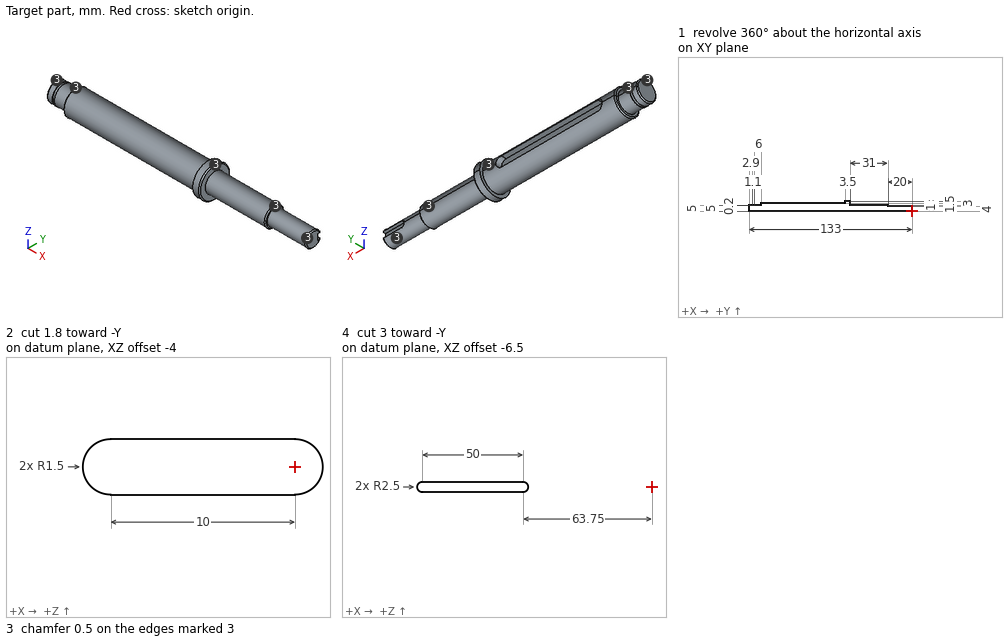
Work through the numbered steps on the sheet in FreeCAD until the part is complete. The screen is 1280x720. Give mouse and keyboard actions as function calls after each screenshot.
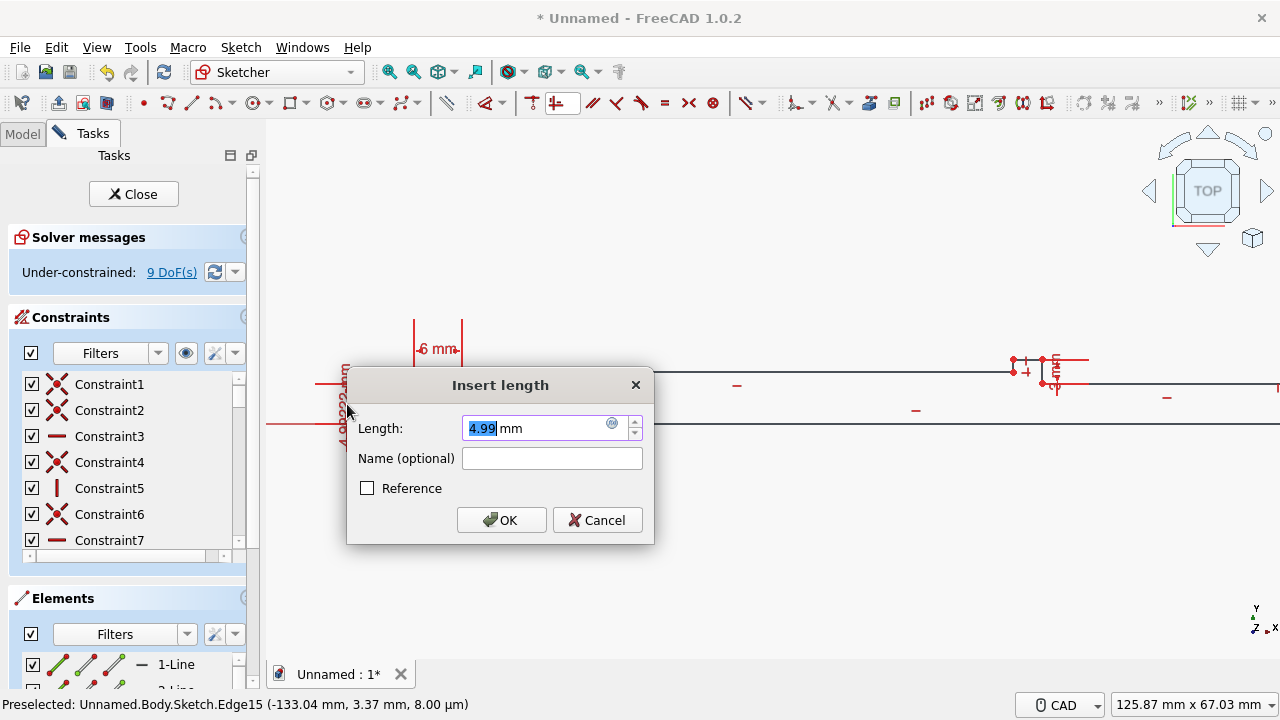
text(5)
key(Return)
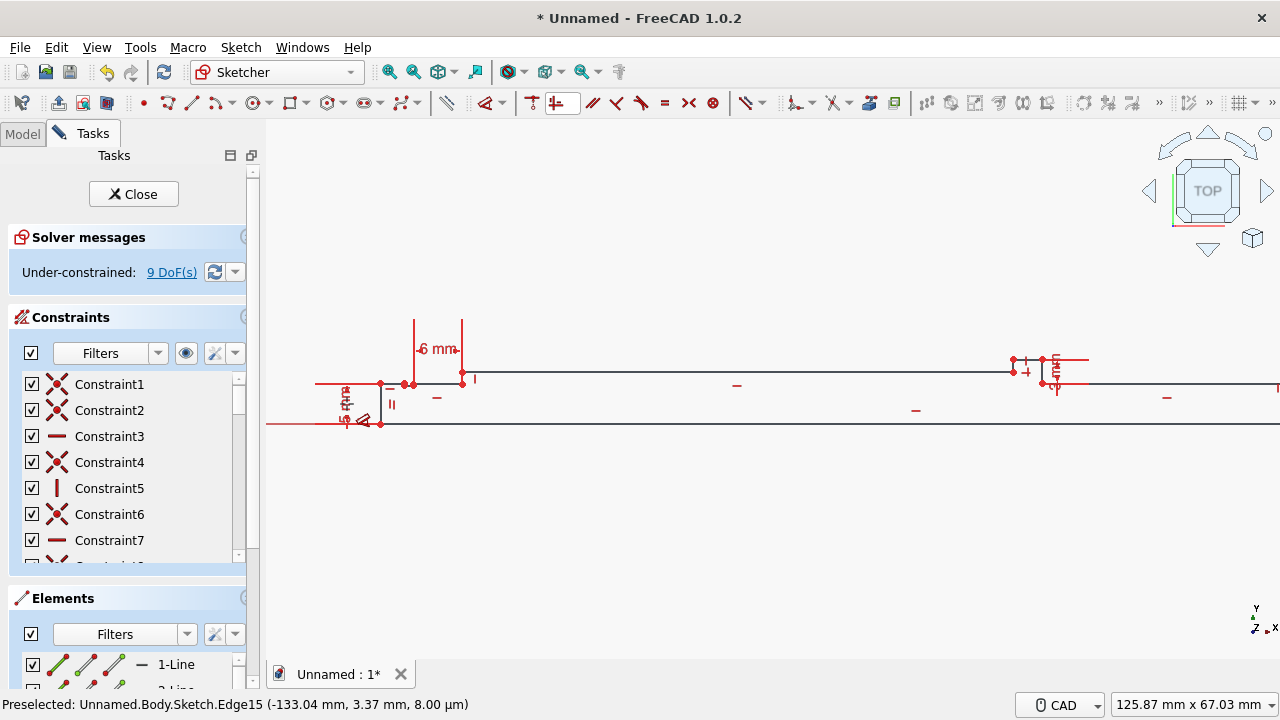
scroll(446, 385, down, 3)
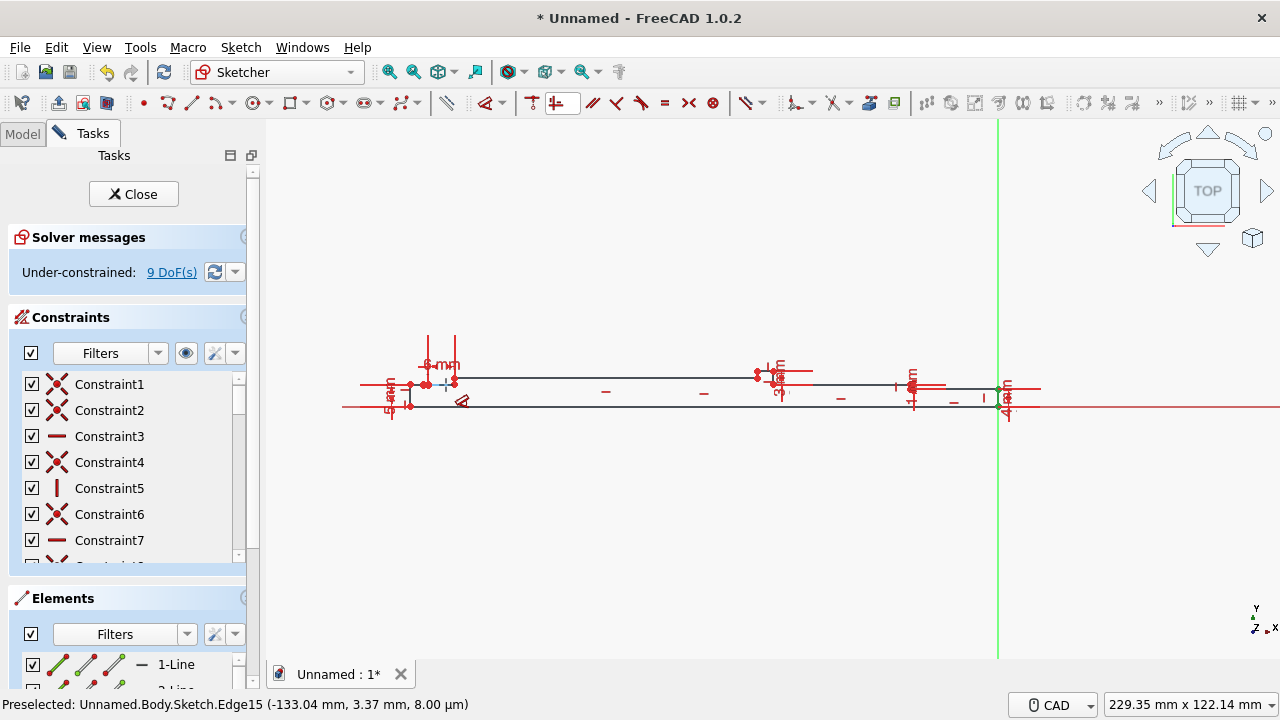
click(972, 389)
click(954, 423)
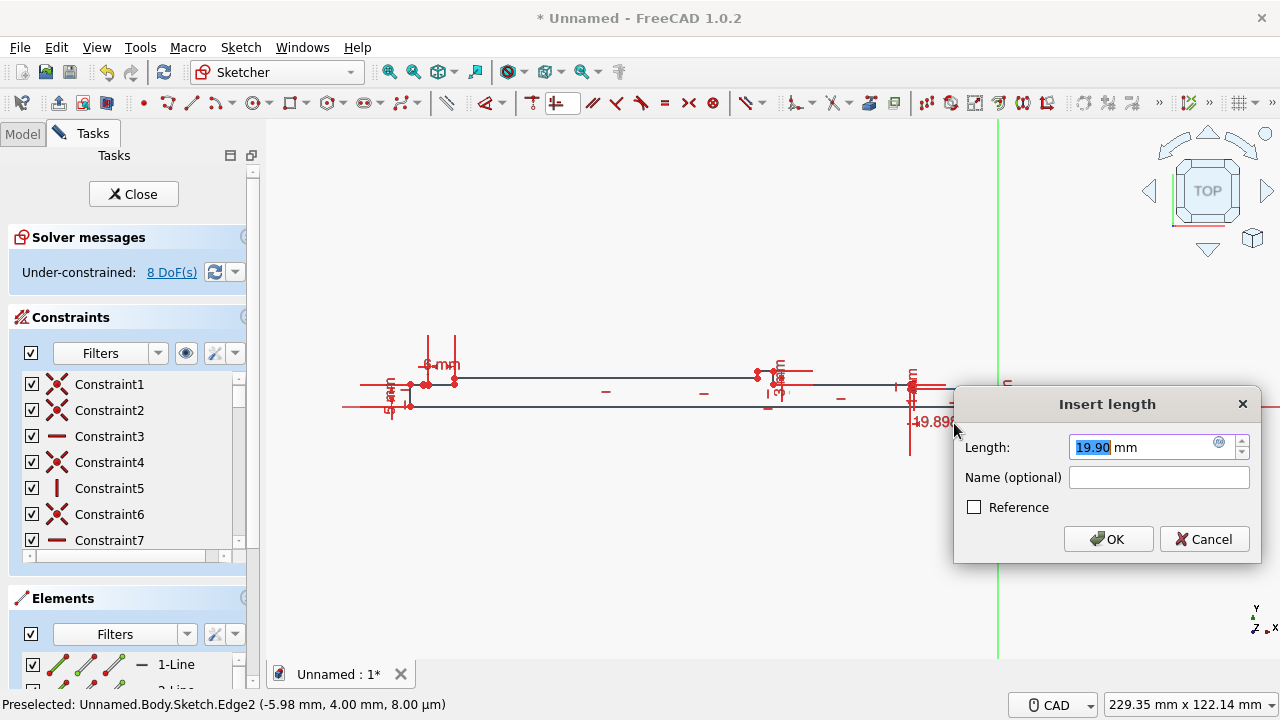
text(20)
key(Return)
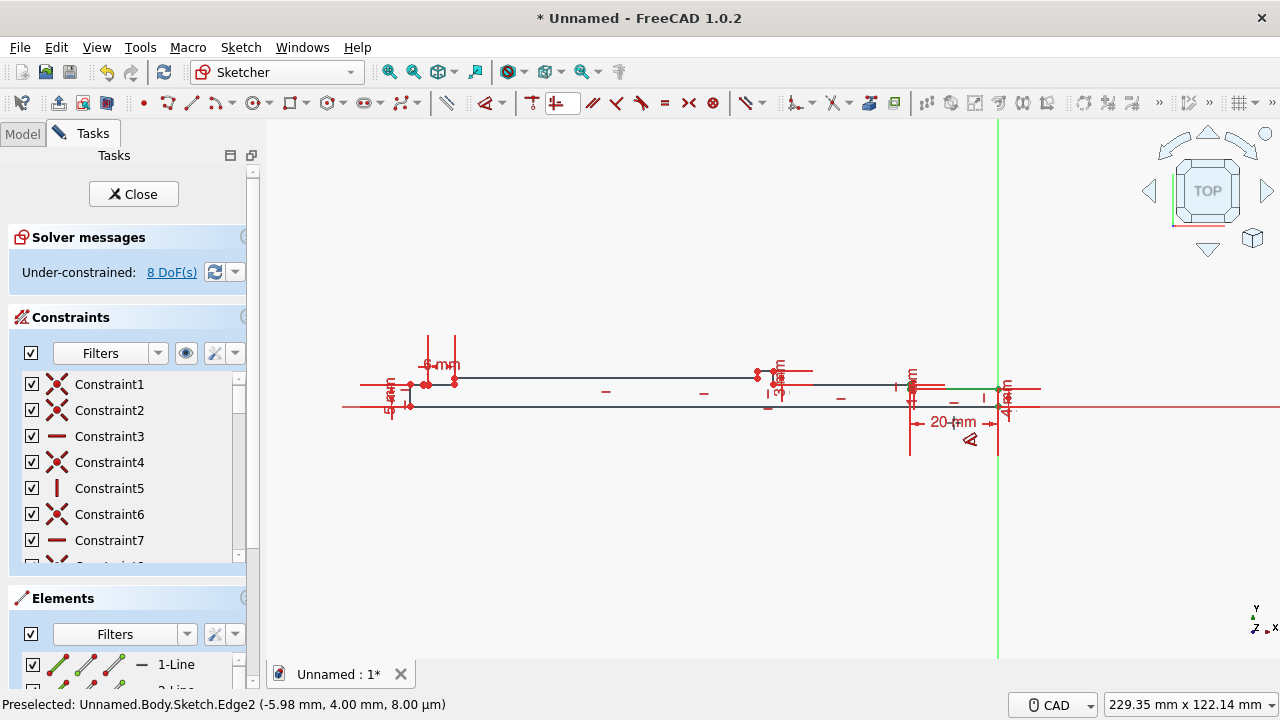
click(869, 385)
click(842, 351)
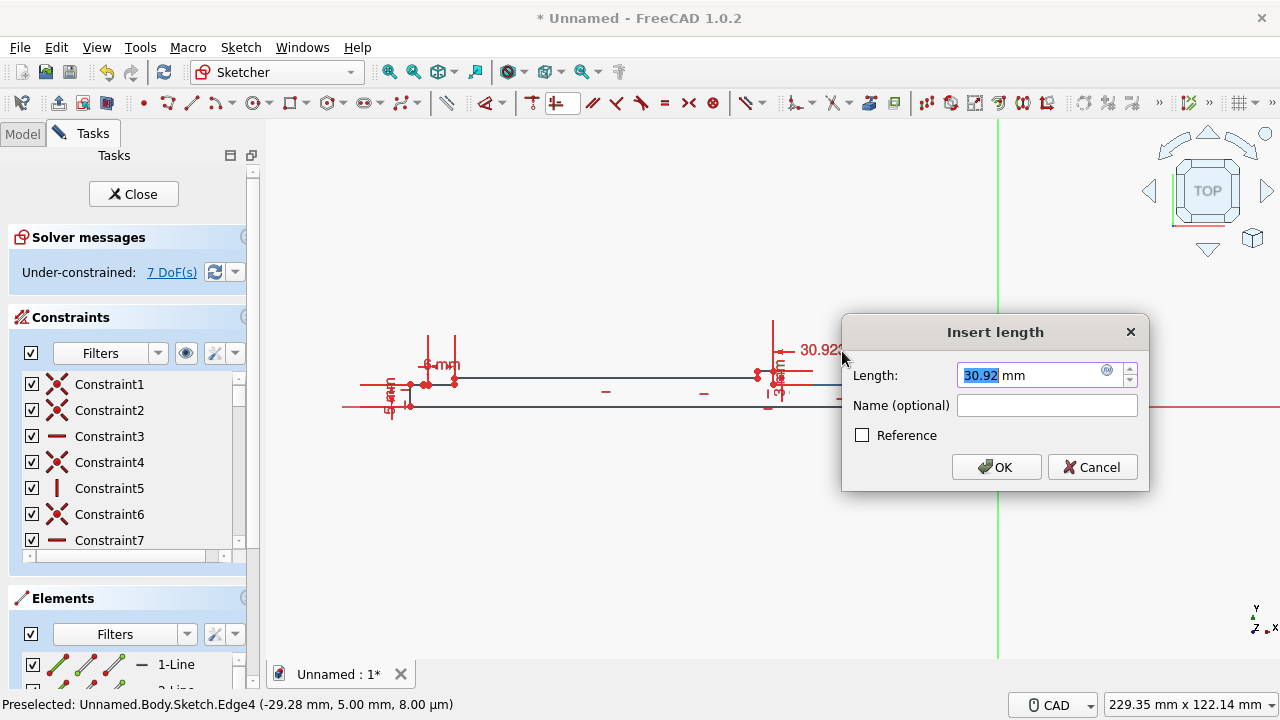
text(31)
key(Return)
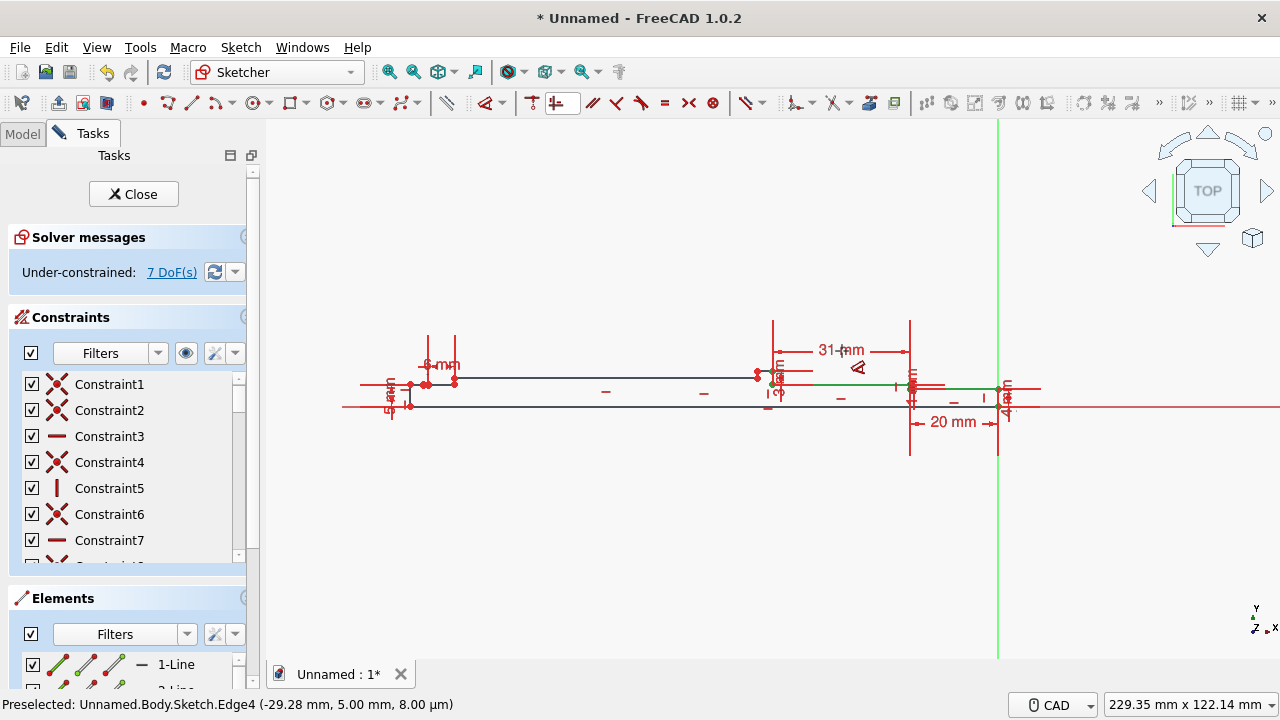
scroll(455, 385, up, 4)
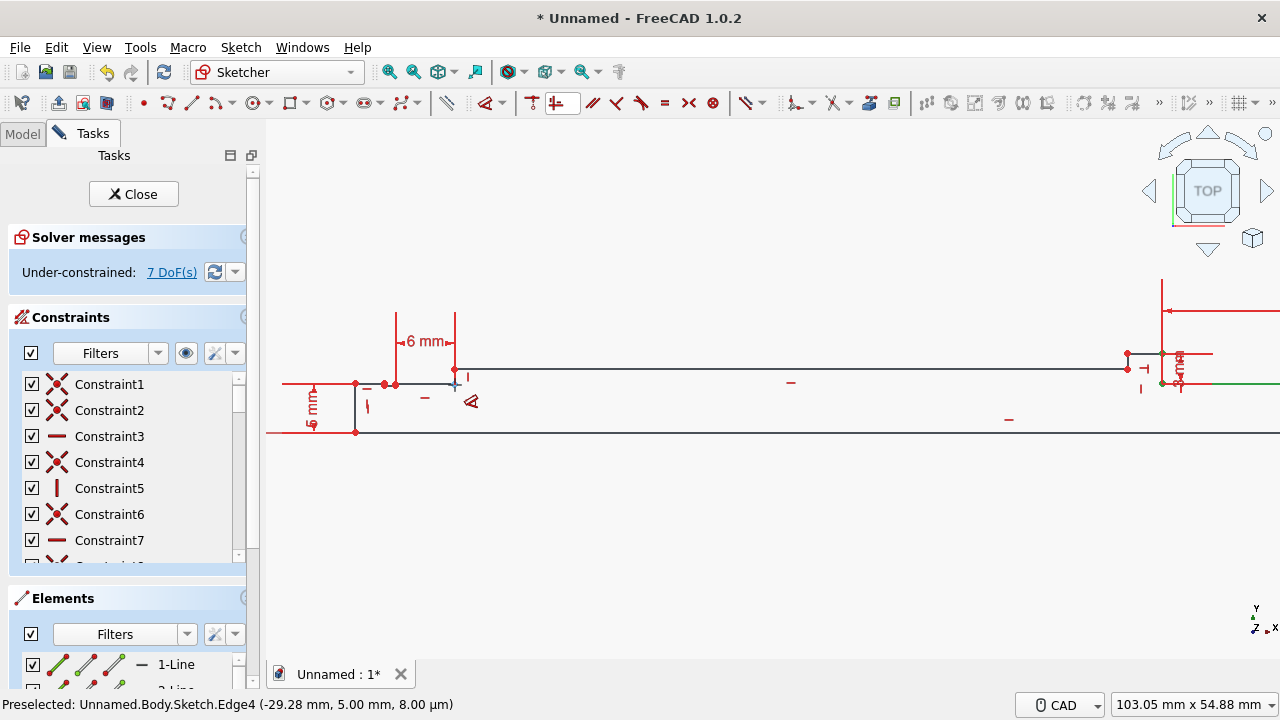
click(455, 384)
click(421, 408)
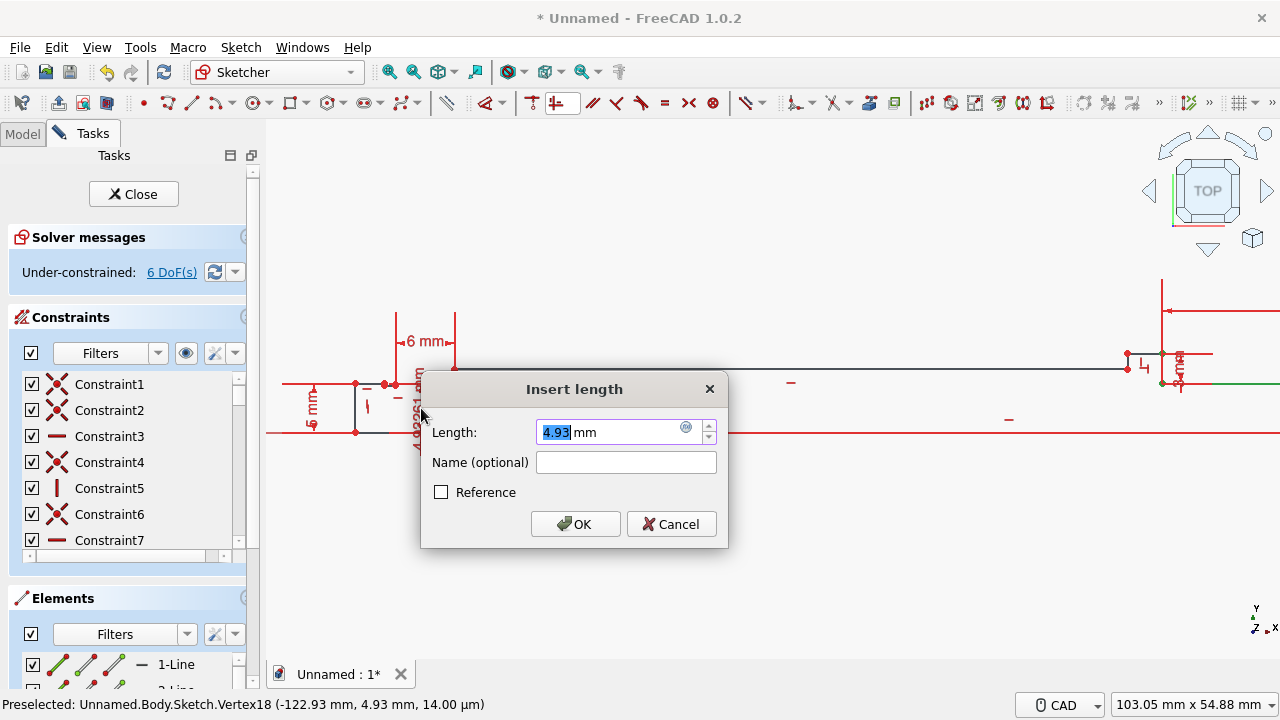
text(5)
key(Return)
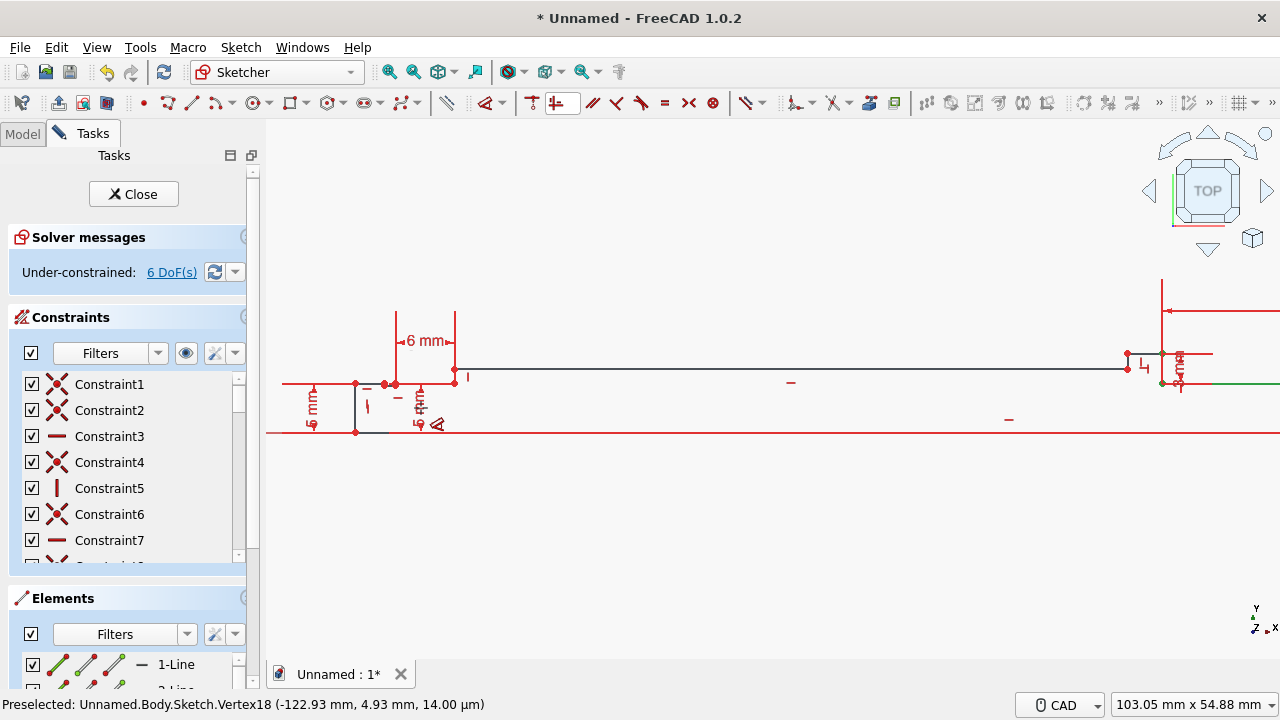
scroll(455, 385, down, 4)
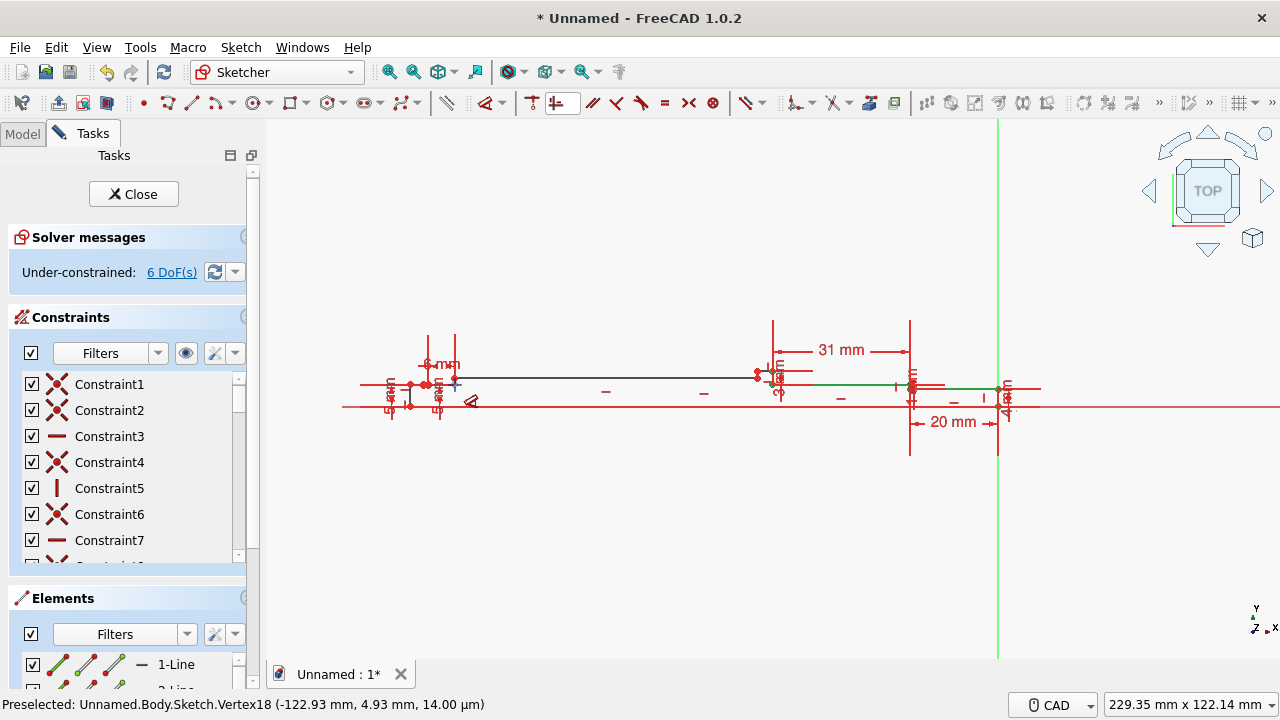
scroll(768, 371, up, 6)